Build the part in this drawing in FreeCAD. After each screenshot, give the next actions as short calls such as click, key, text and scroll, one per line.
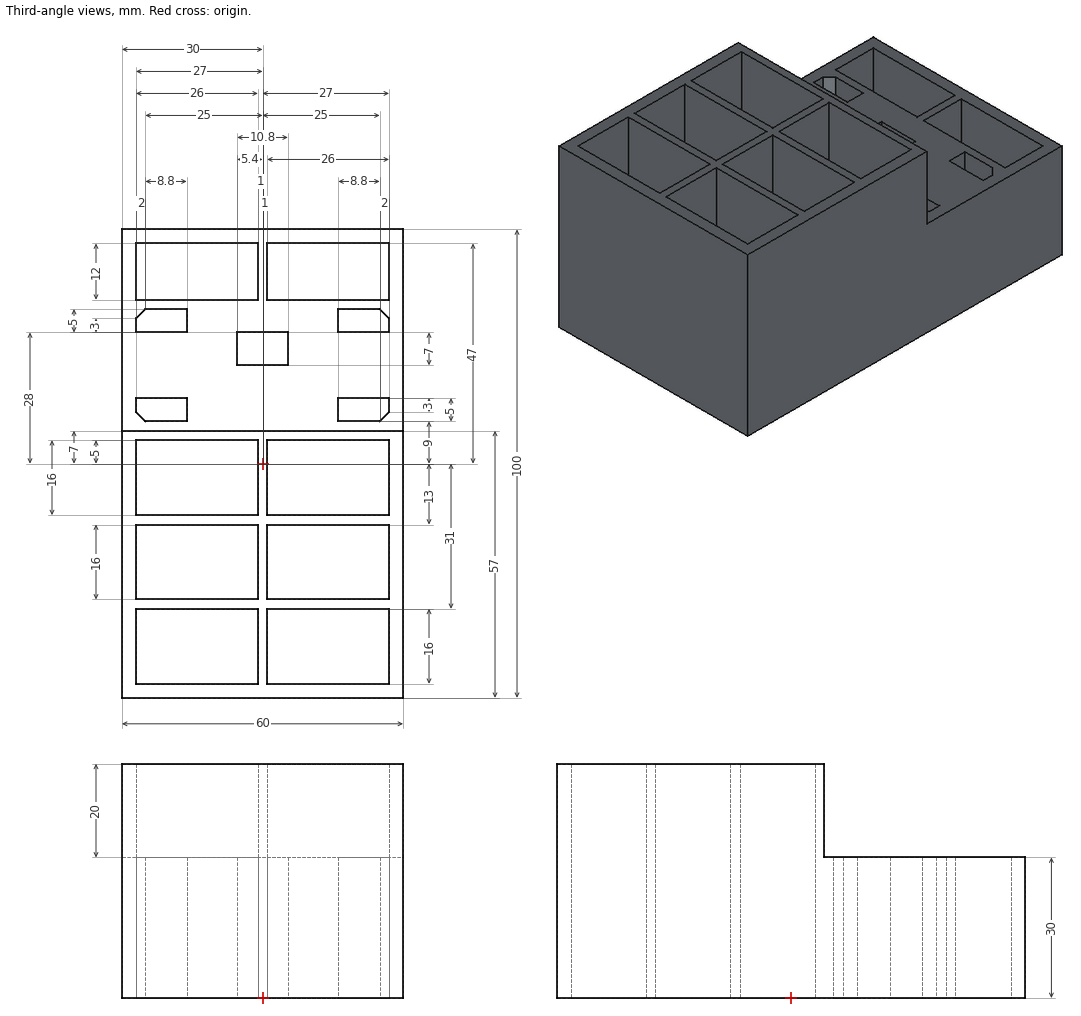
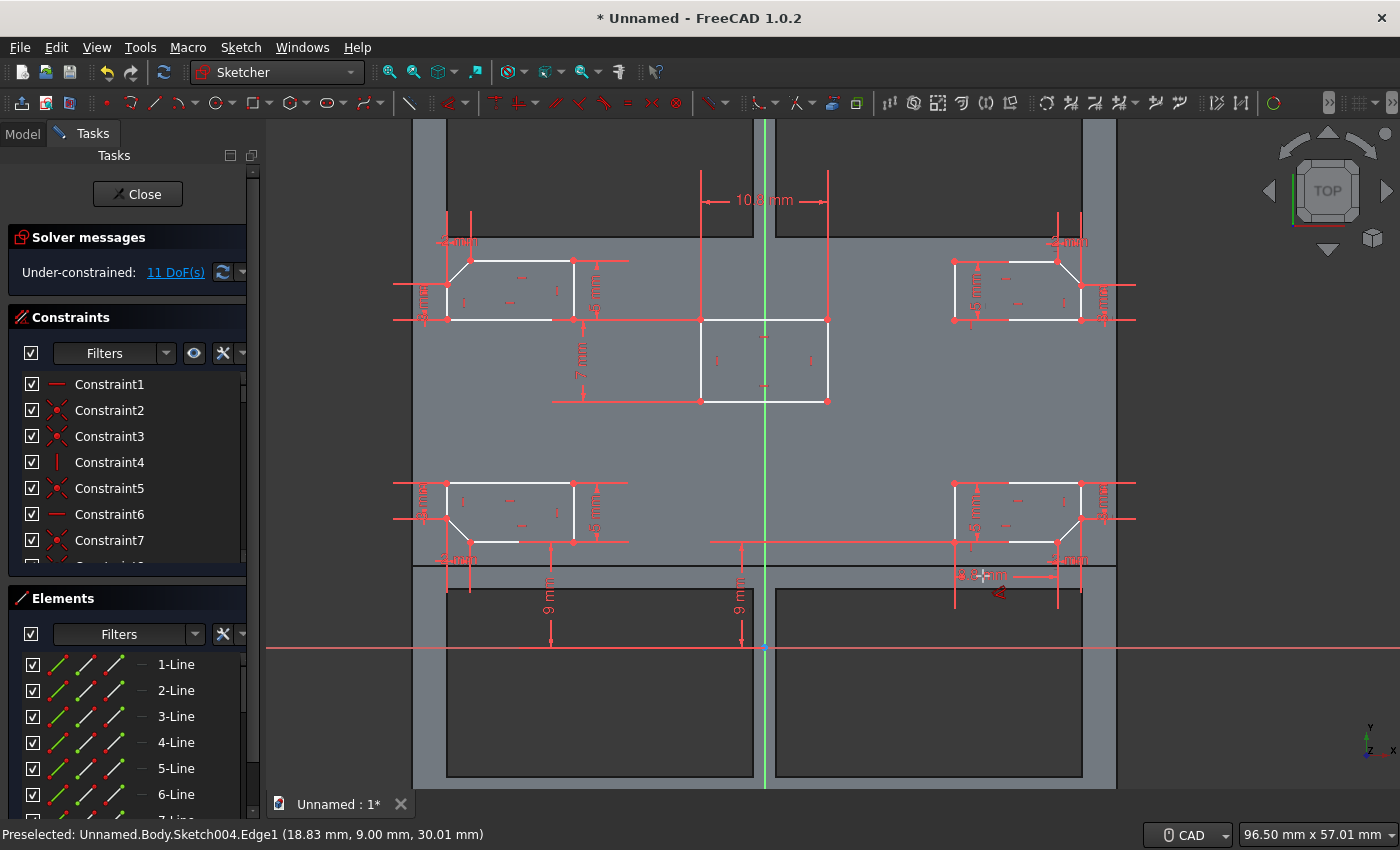
click(543, 261)
click(546, 227)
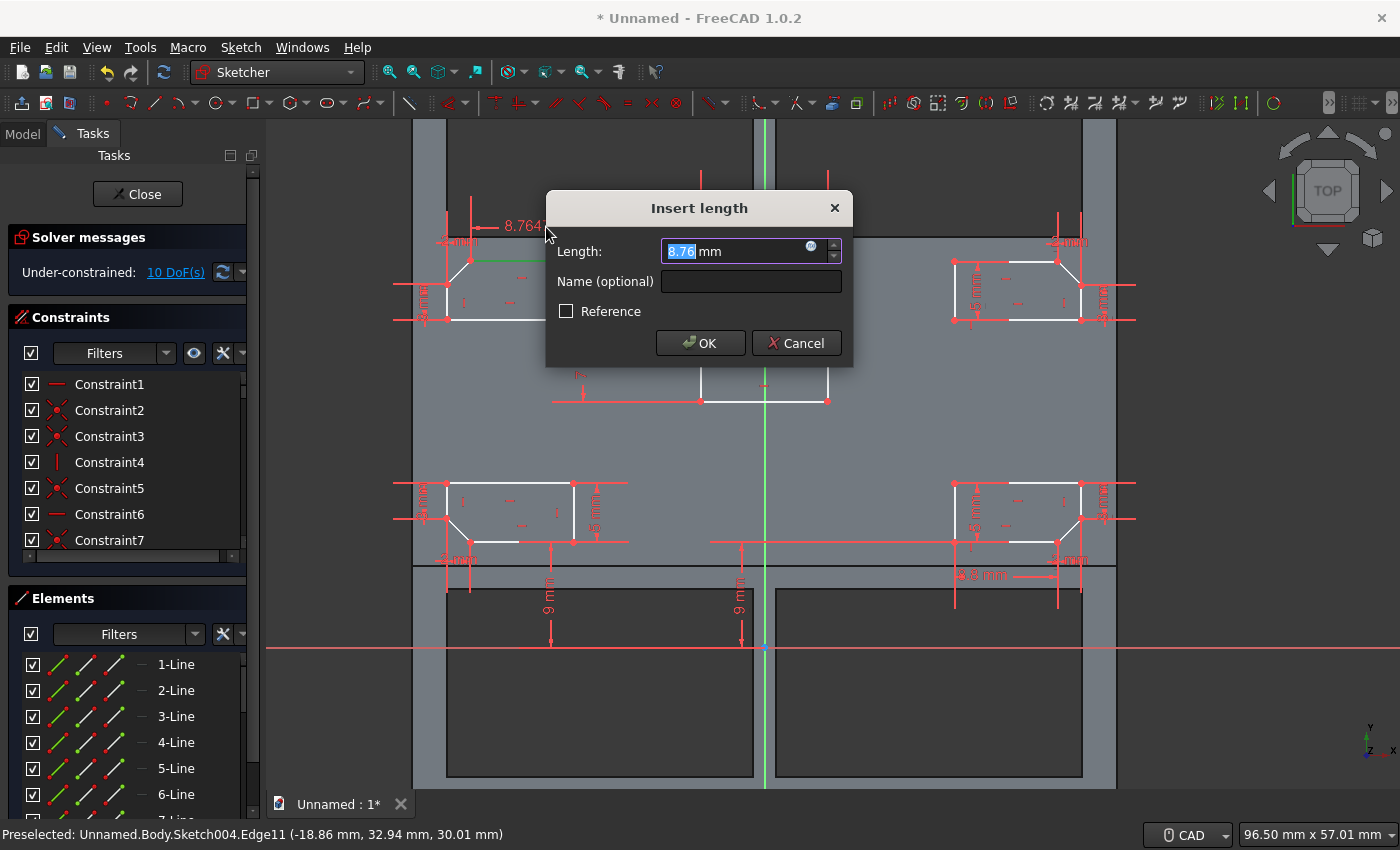
text(8.8)
key(Return)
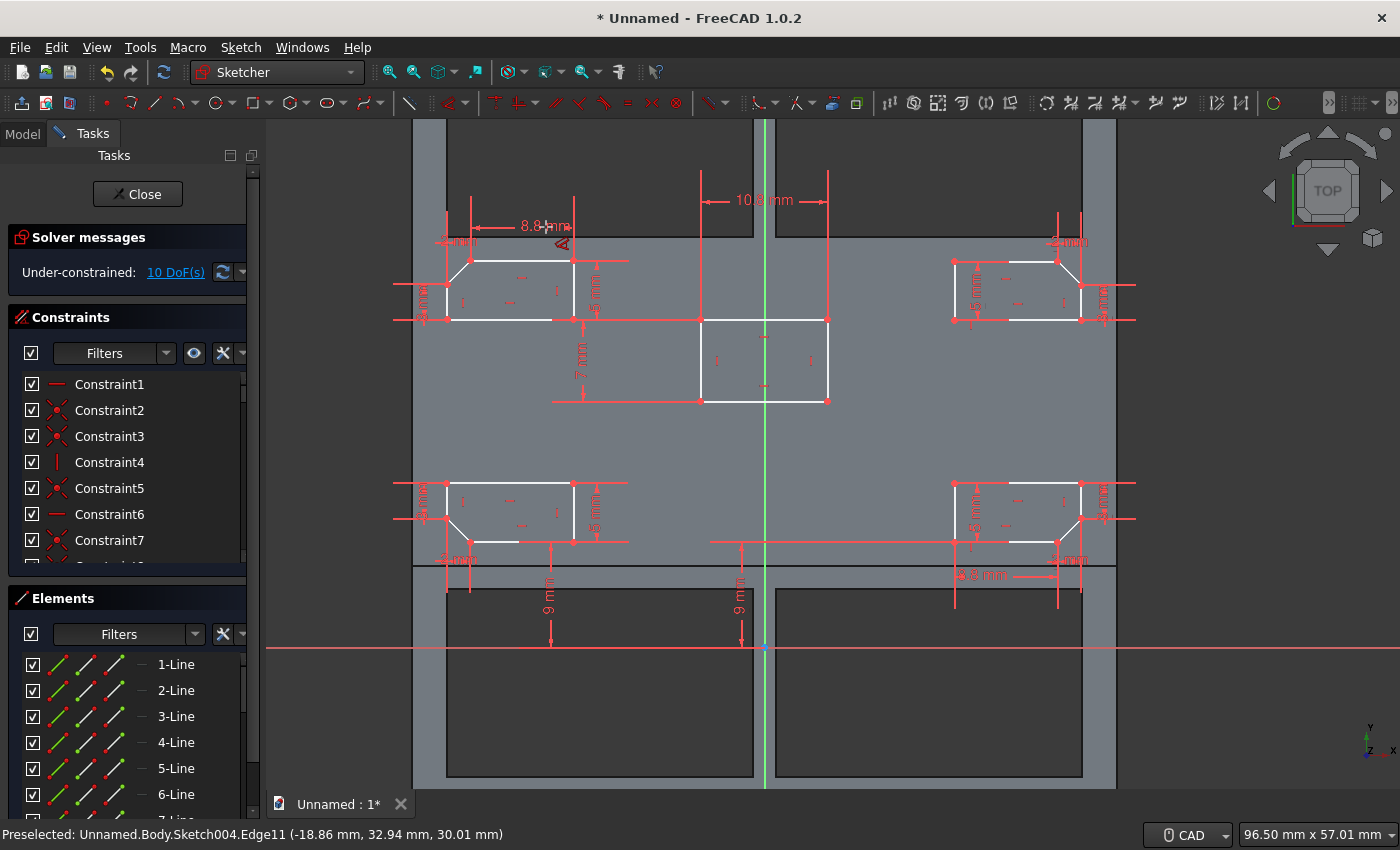
click(1027, 262)
click(983, 228)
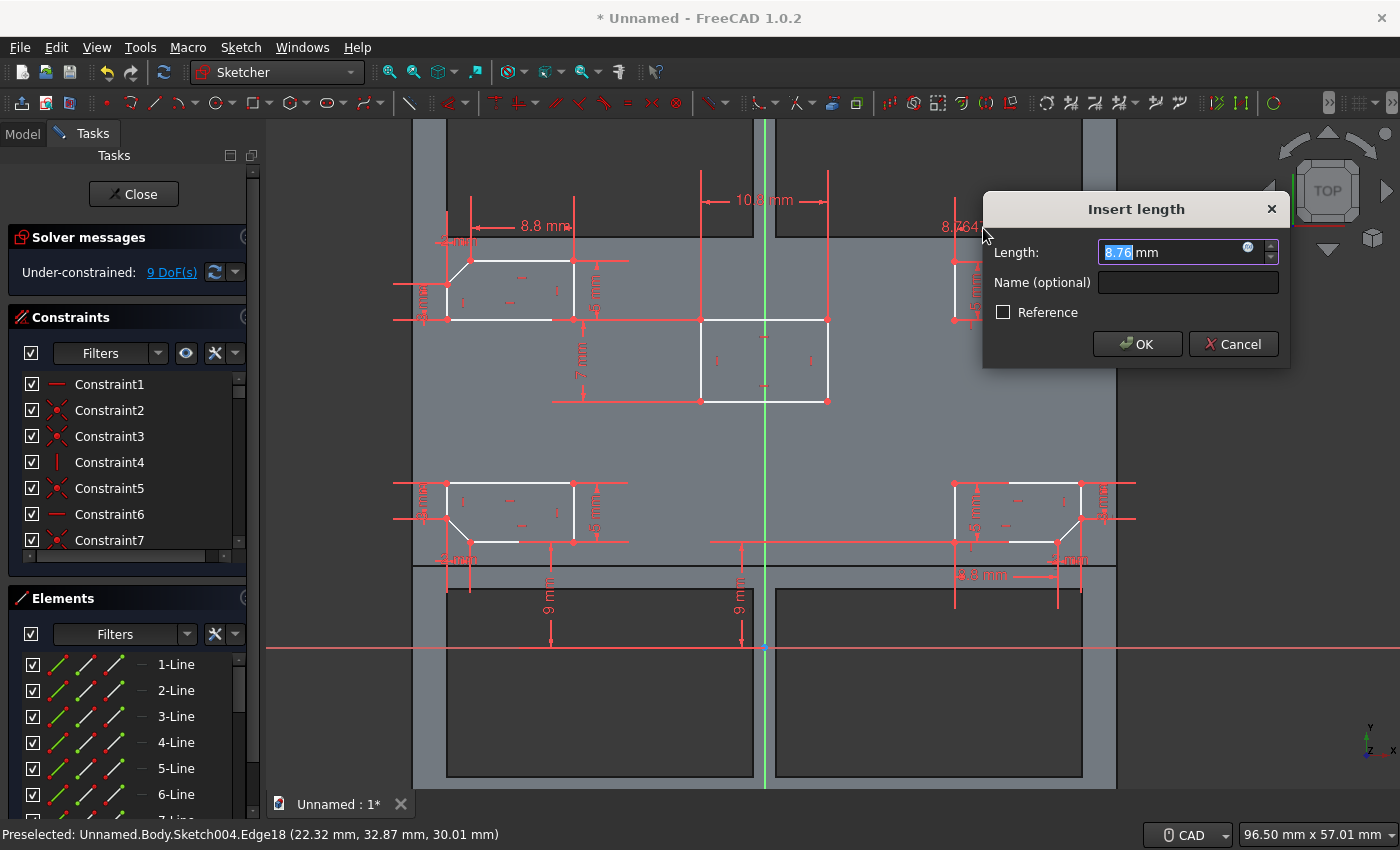
text(8.8)
key(Return)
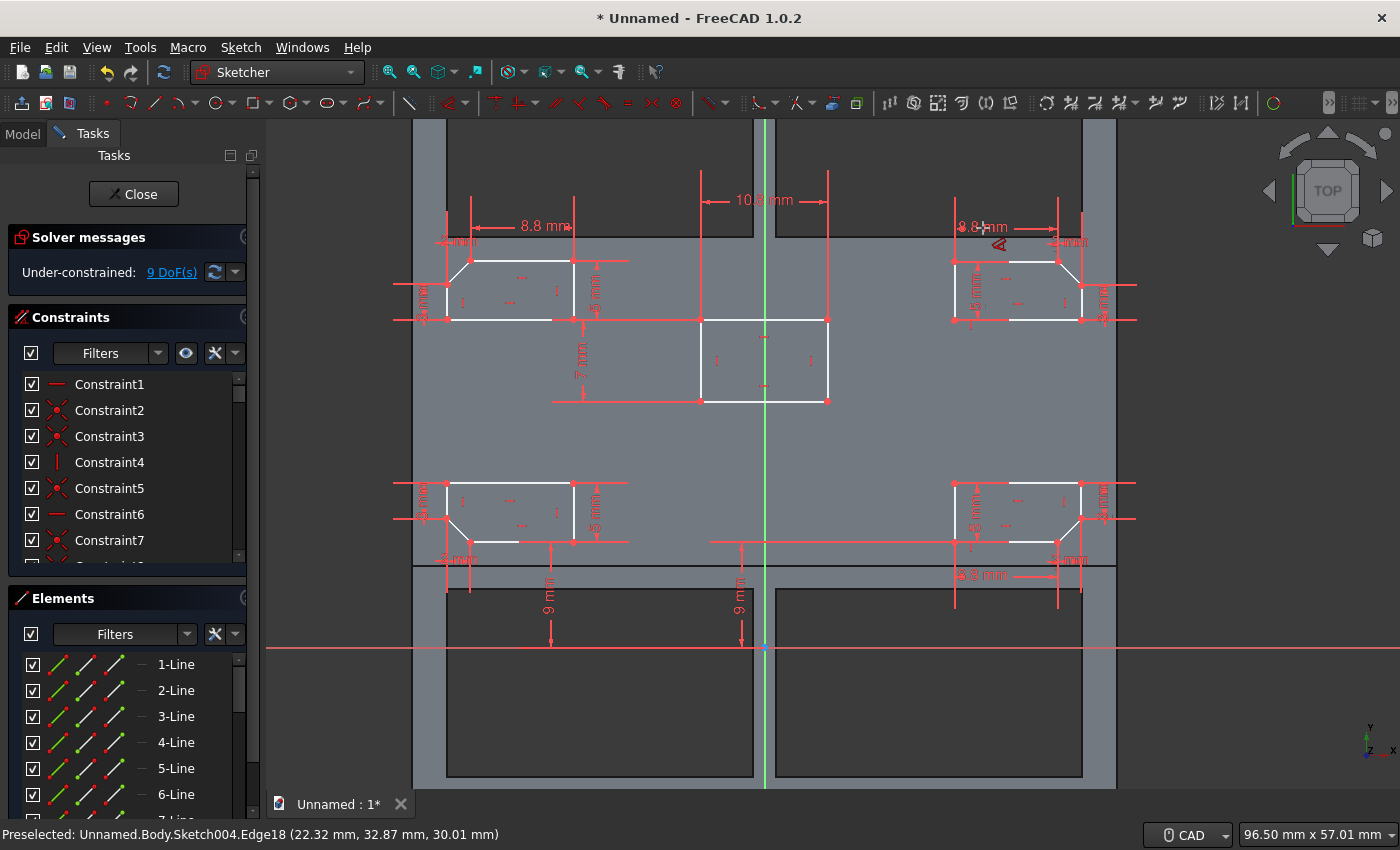
click(502, 542)
click(522, 508)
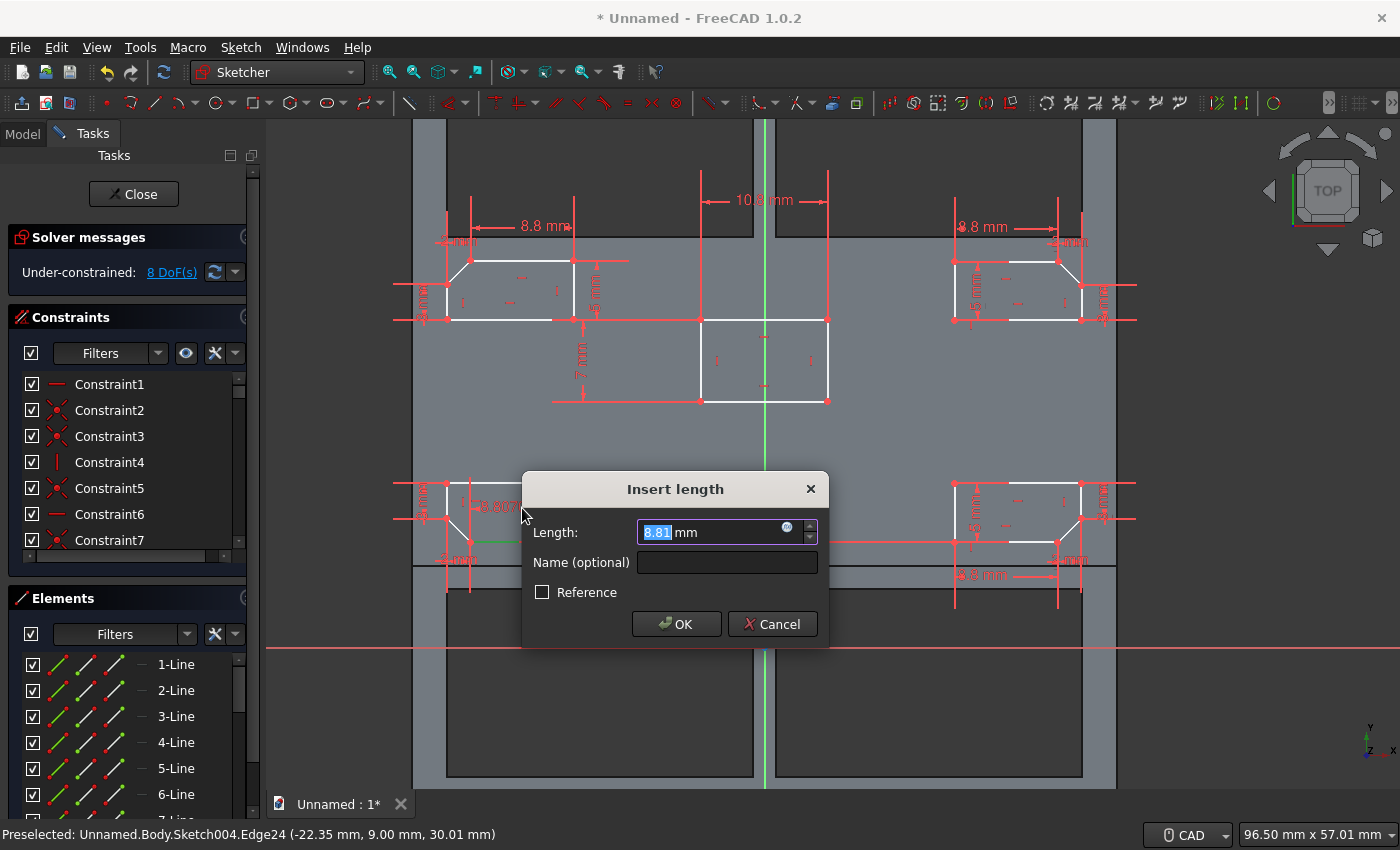
text(8.8)
key(Return)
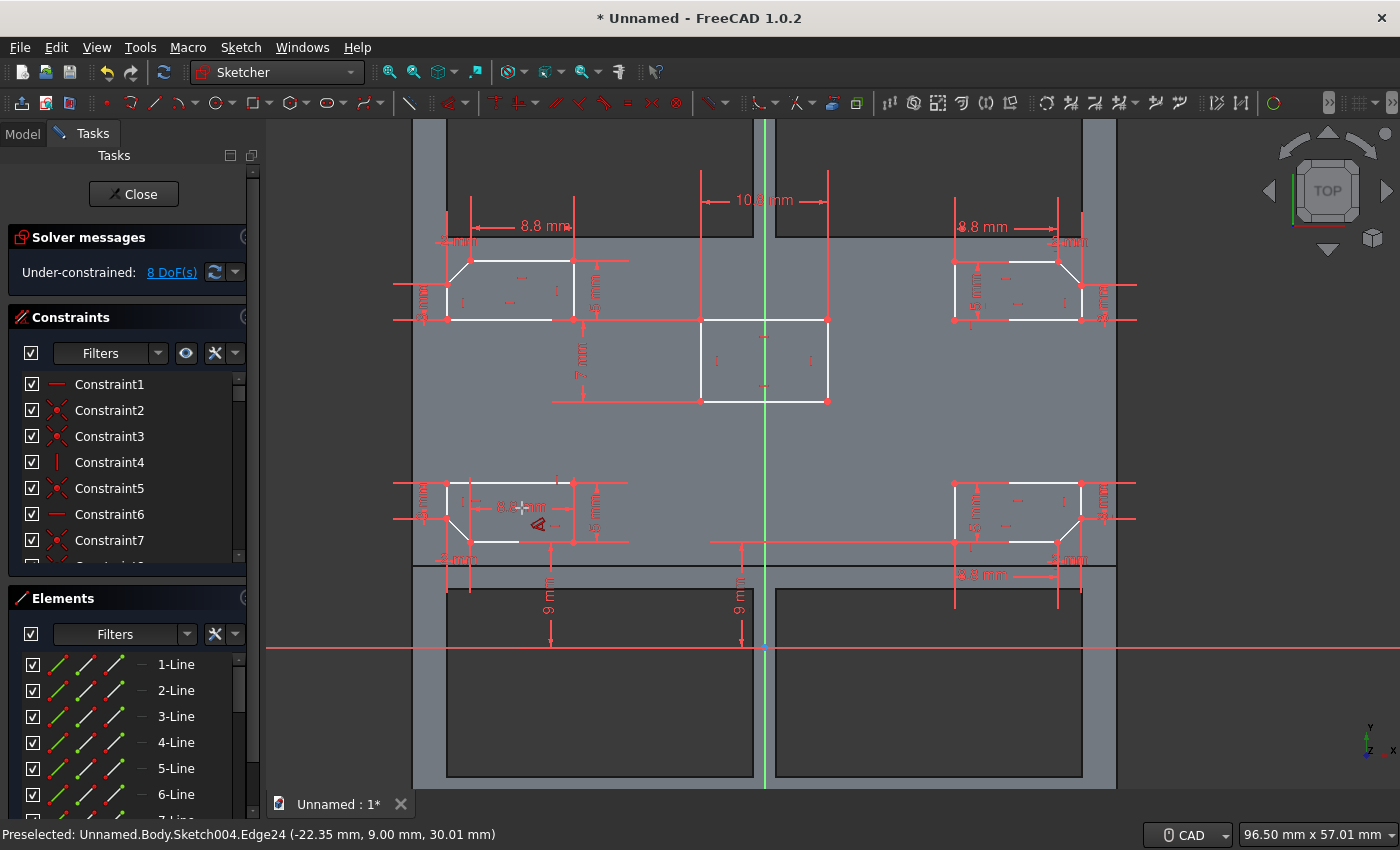
click(1058, 542)
click(911, 682)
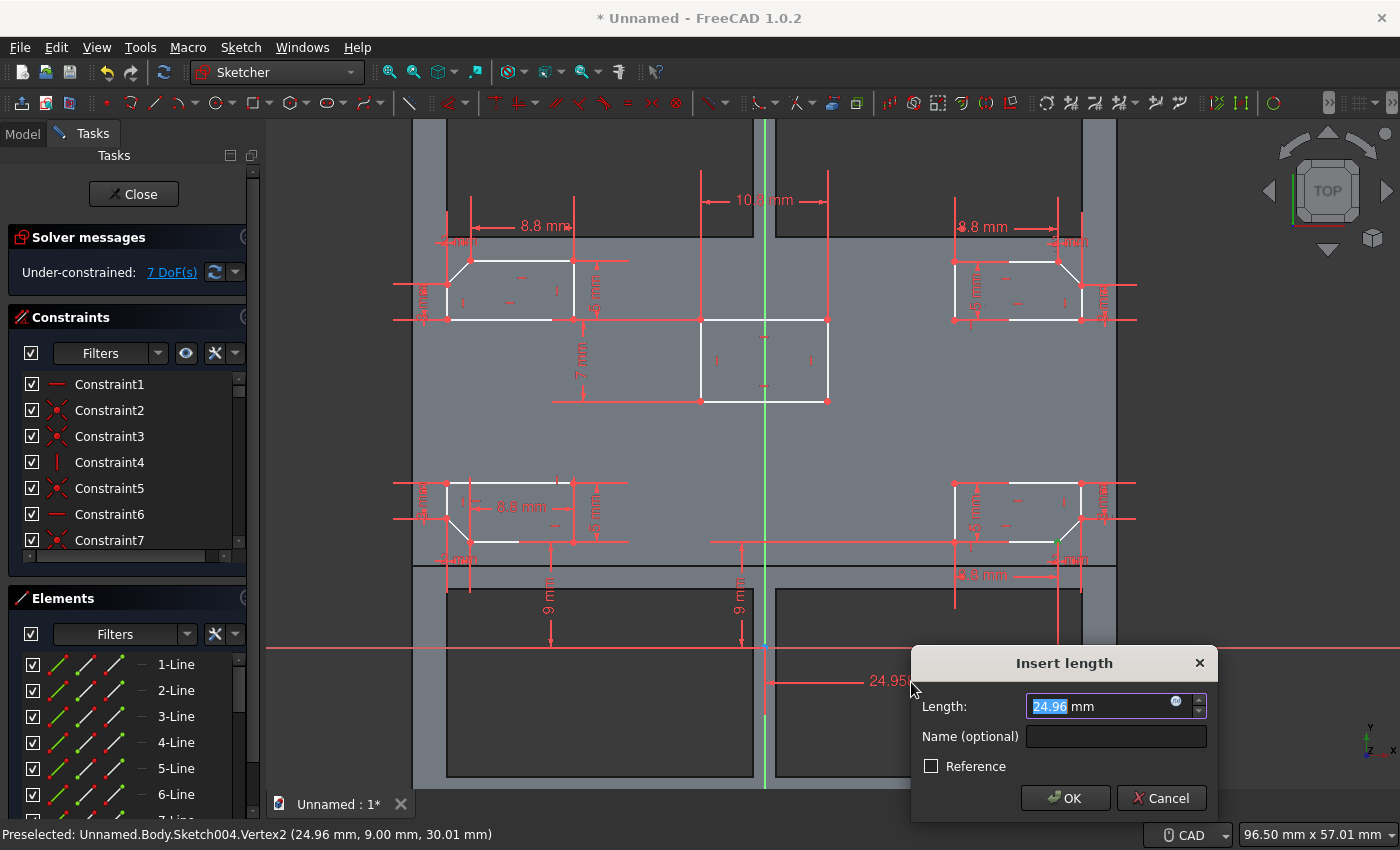
text(25)
key(Return)